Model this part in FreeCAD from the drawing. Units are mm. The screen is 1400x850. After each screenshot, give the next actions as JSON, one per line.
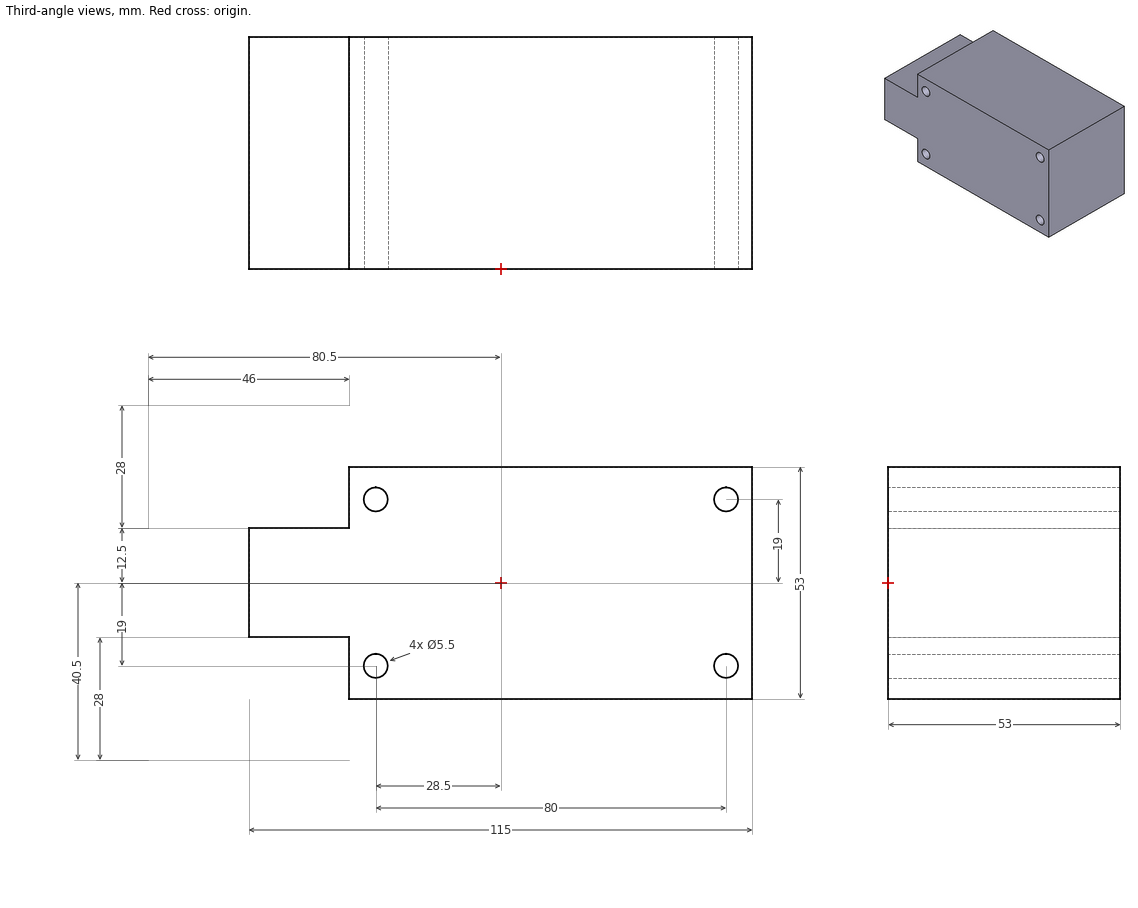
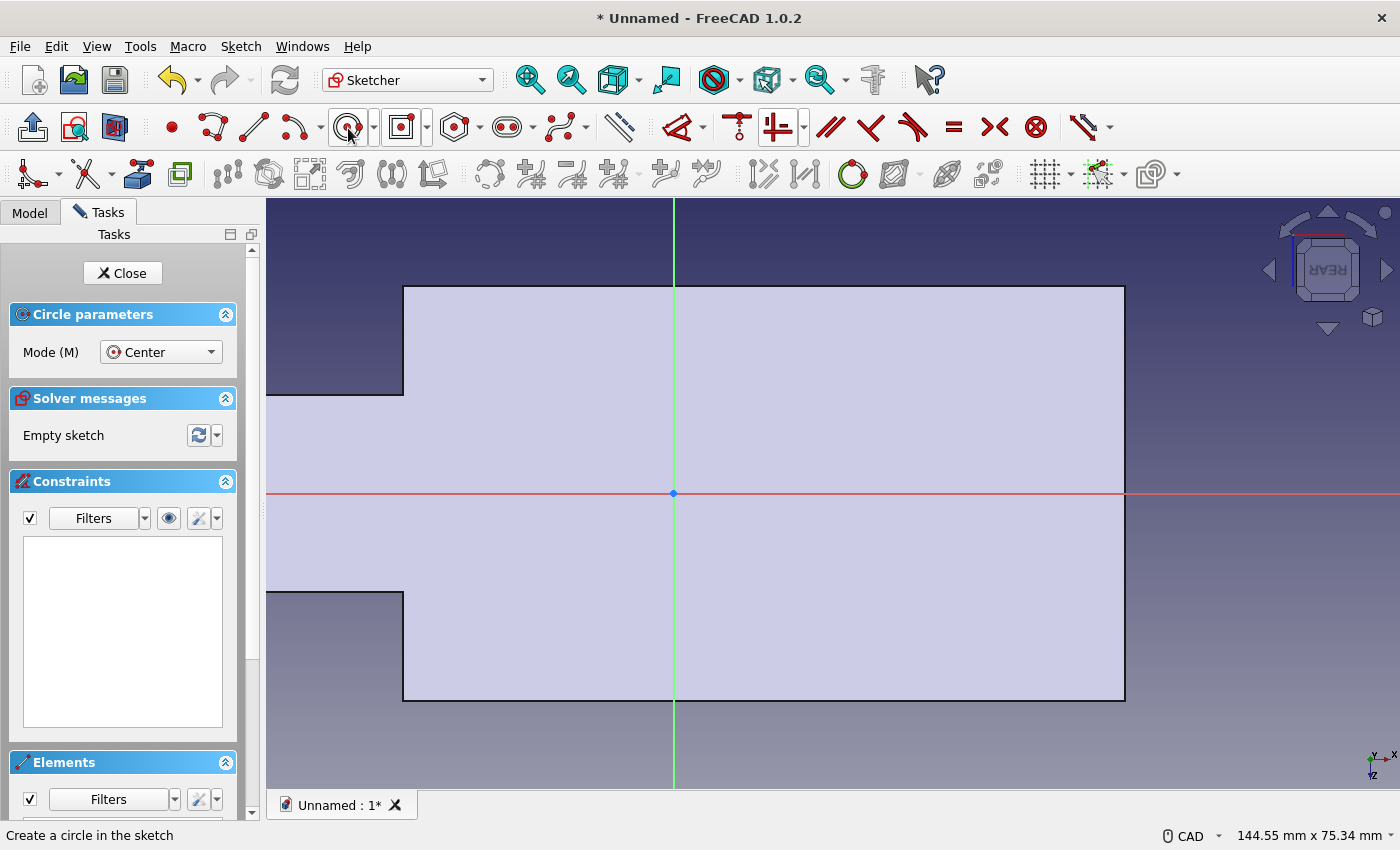
{"action": "left_click", "coordinate": [450, 344]}
{"action": "mouse_move", "coordinate": [465, 329]}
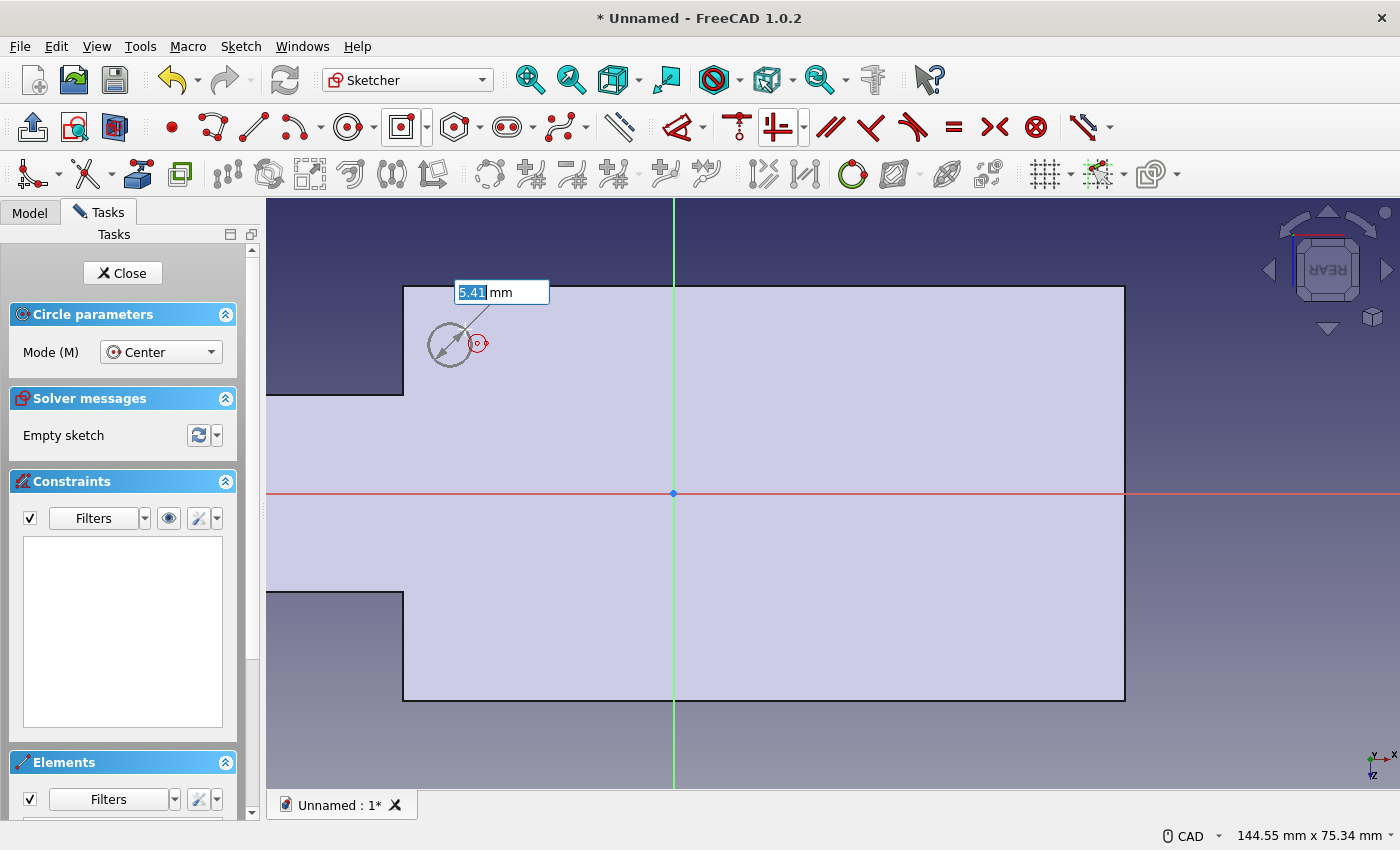
{"action": "type", "text": "5.5"}
{"action": "key", "text": "Return"}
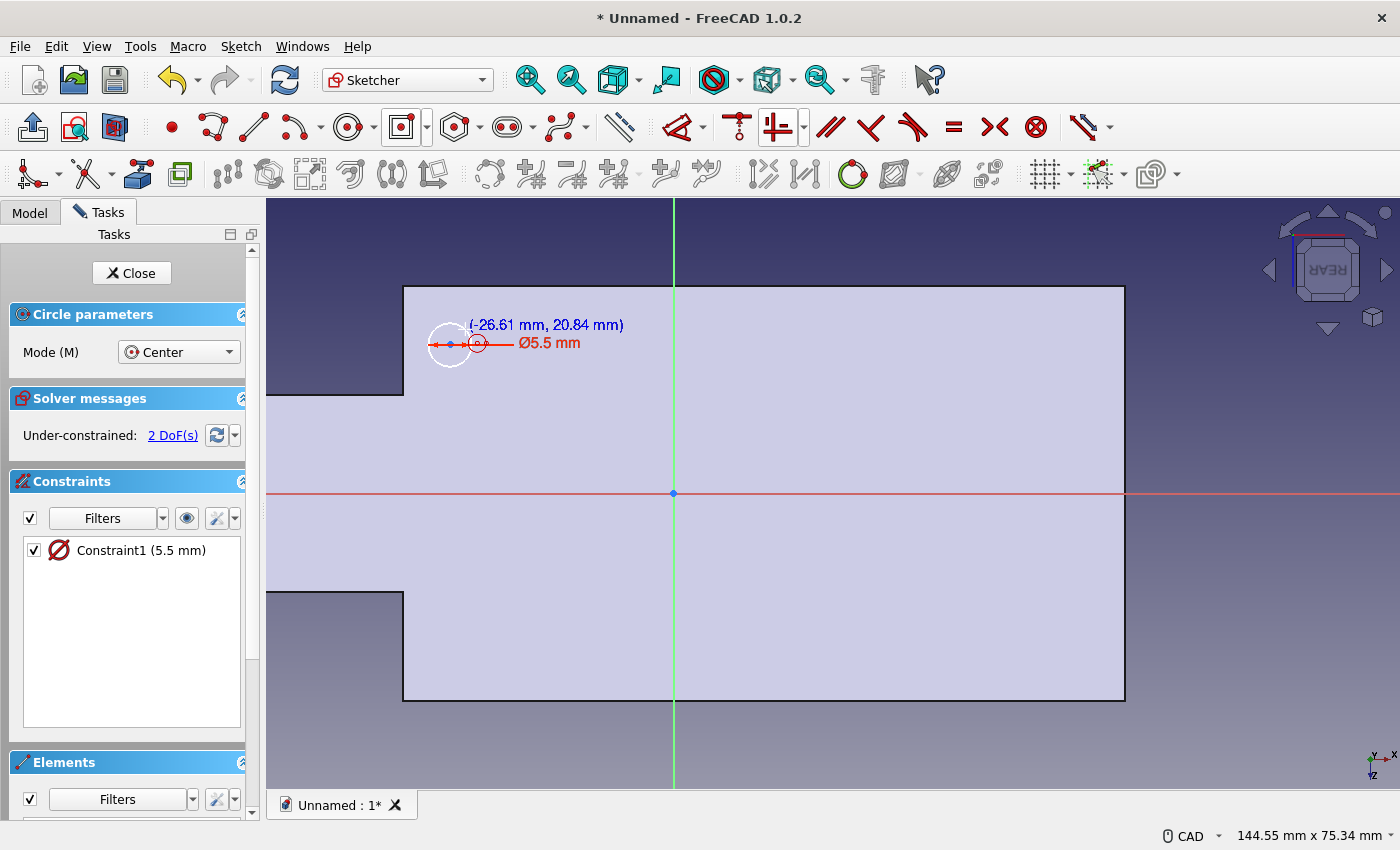
{"action": "left_click", "coordinate": [1078, 344]}
{"action": "mouse_move", "coordinate": [1093, 329]}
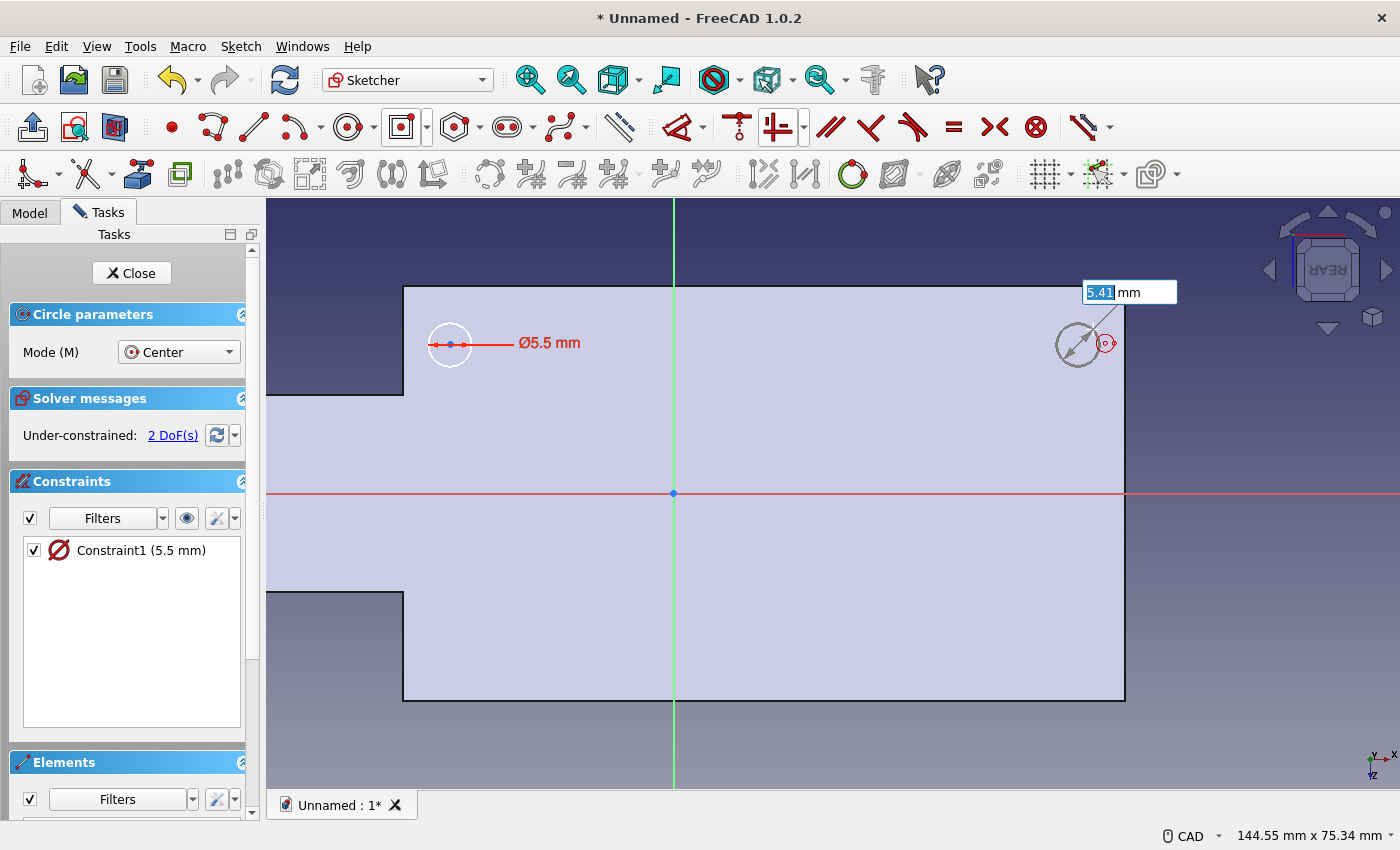
{"action": "type", "text": "5.5"}
{"action": "key", "text": "Return"}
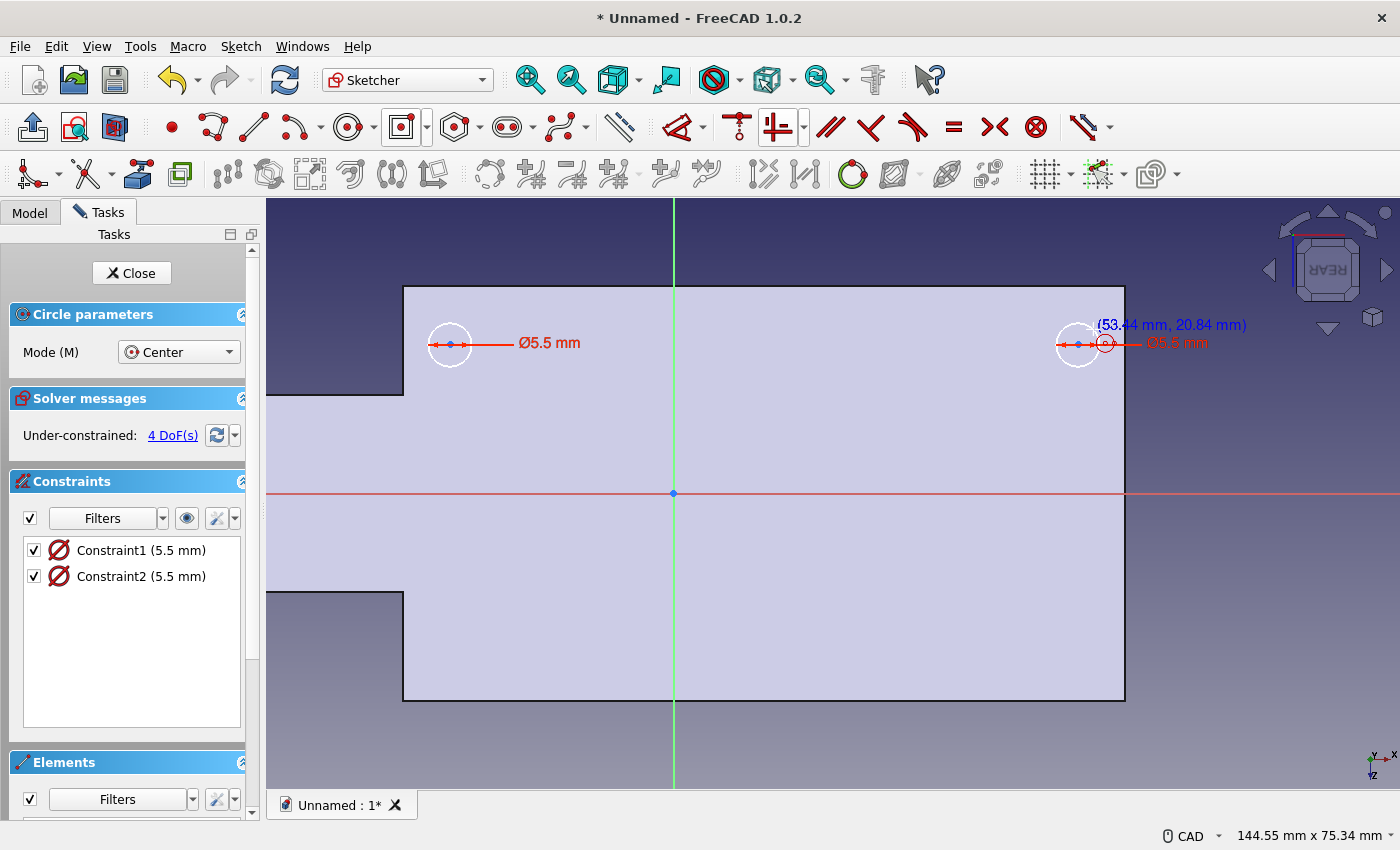
{"action": "left_click", "coordinate": [1078, 643]}
{"action": "mouse_move", "coordinate": [1093, 627]}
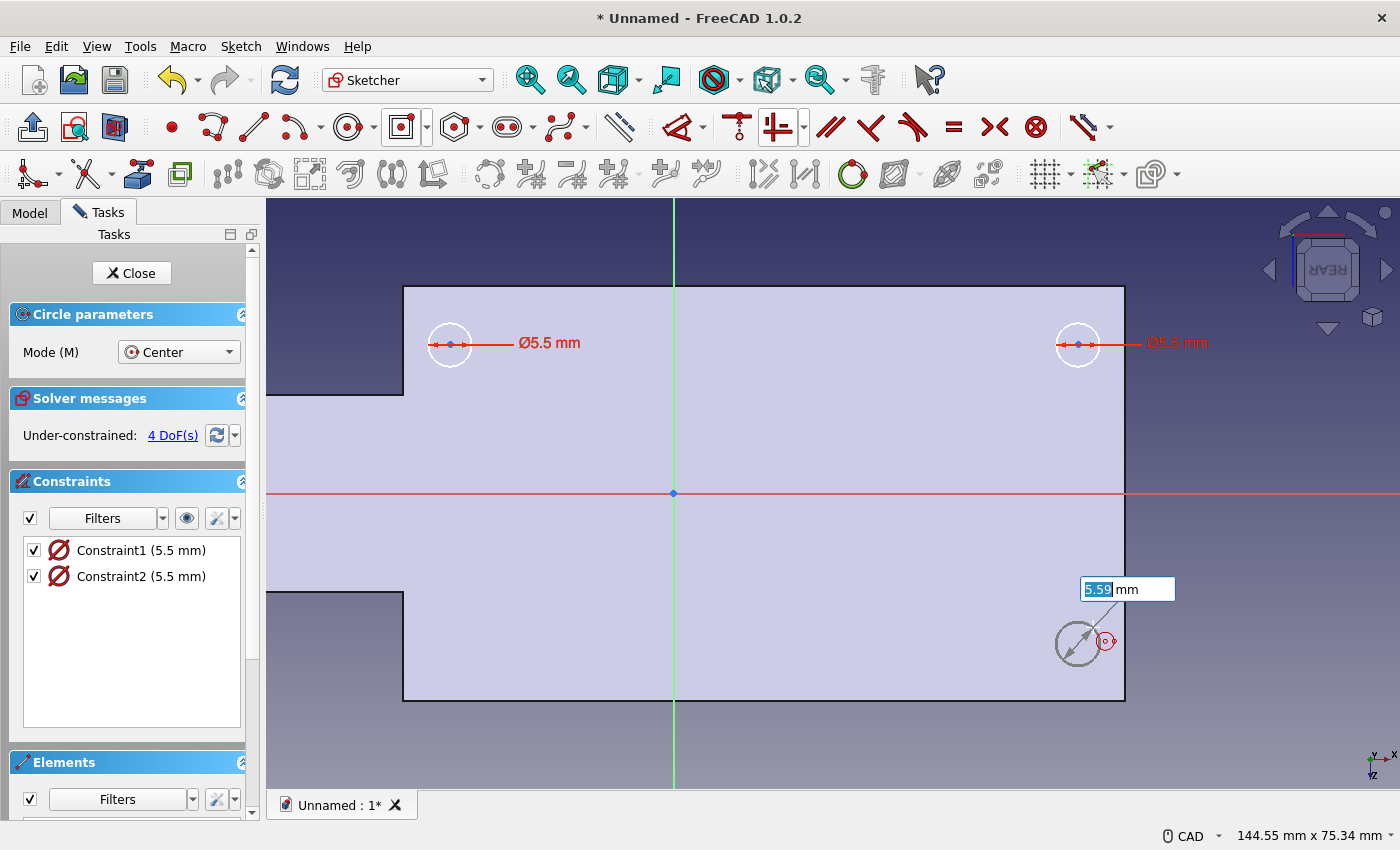
{"action": "type", "text": "5.5"}
{"action": "key", "text": "Return"}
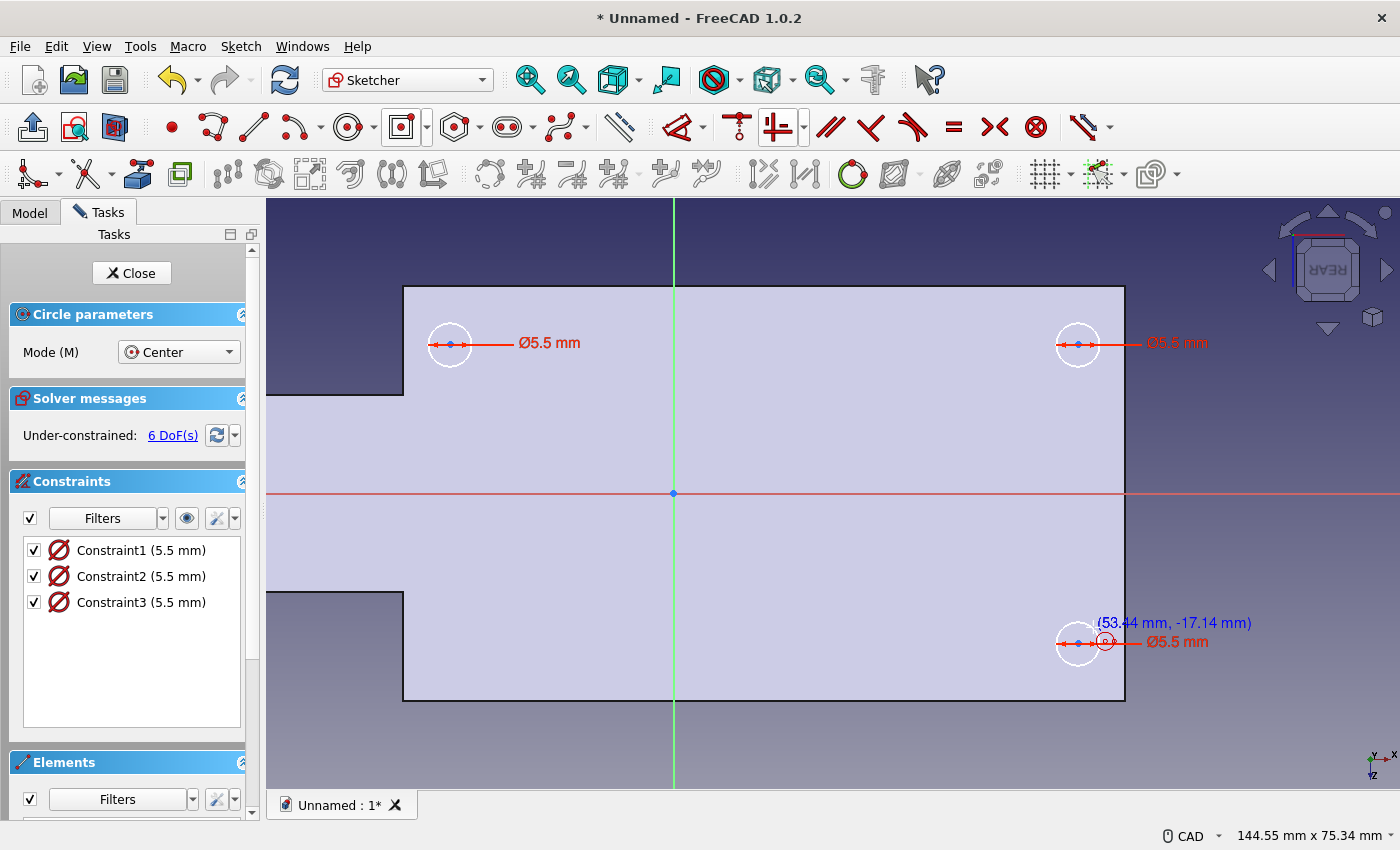
{"action": "left_click", "coordinate": [450, 643]}
{"action": "mouse_move", "coordinate": [465, 627]}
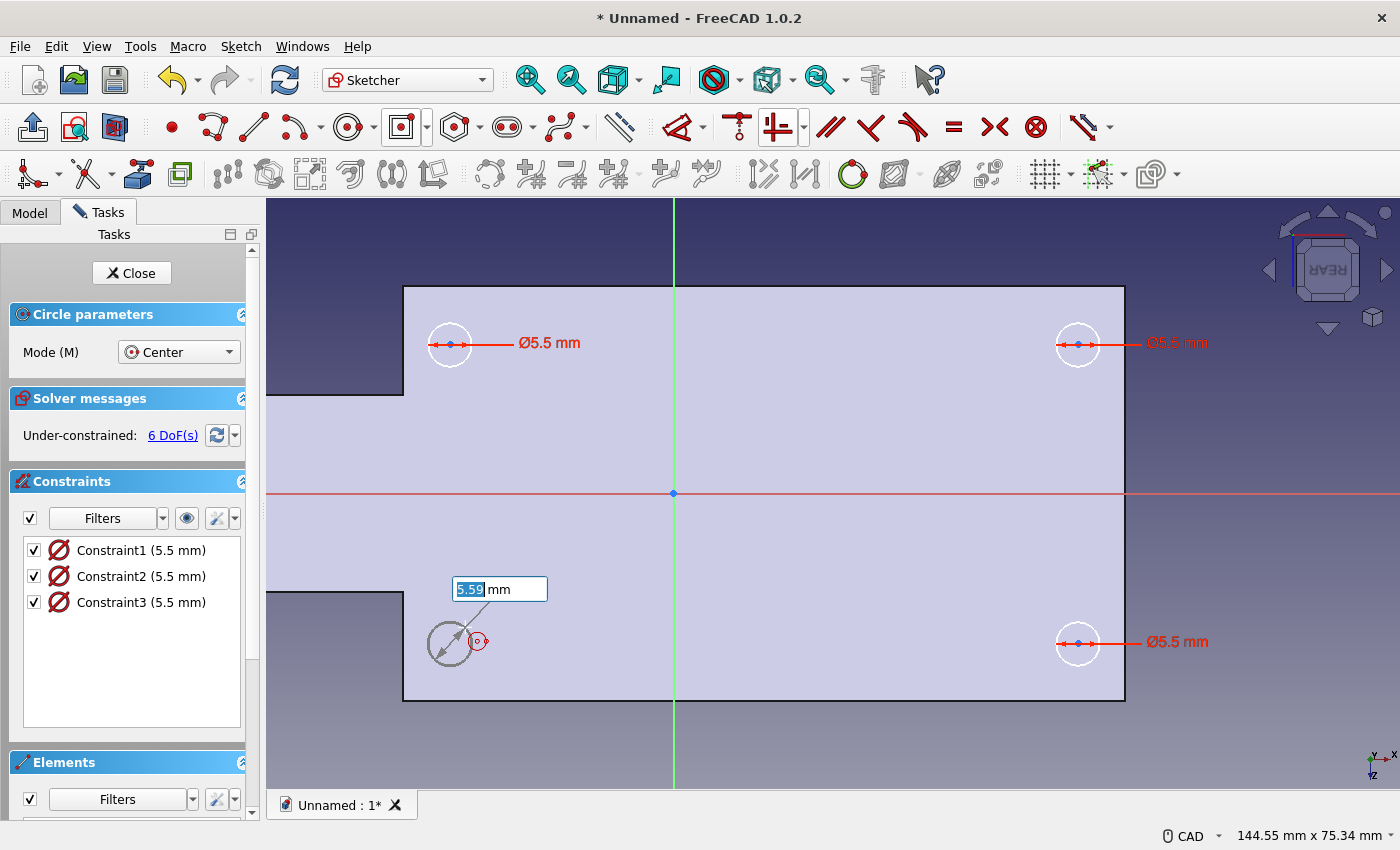
{"action": "type", "text": "5.5"}
{"action": "key", "text": "Return"}
{"action": "key", "text": "Escape"}